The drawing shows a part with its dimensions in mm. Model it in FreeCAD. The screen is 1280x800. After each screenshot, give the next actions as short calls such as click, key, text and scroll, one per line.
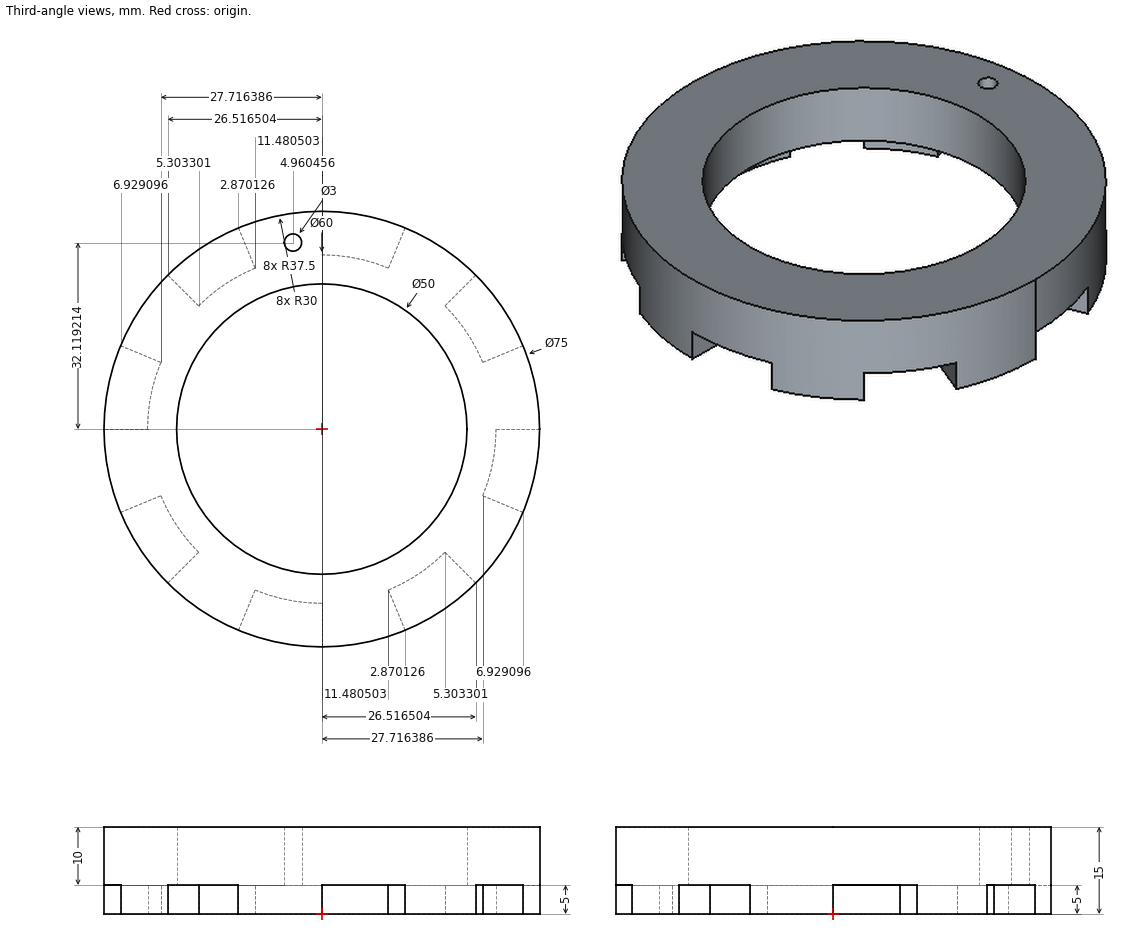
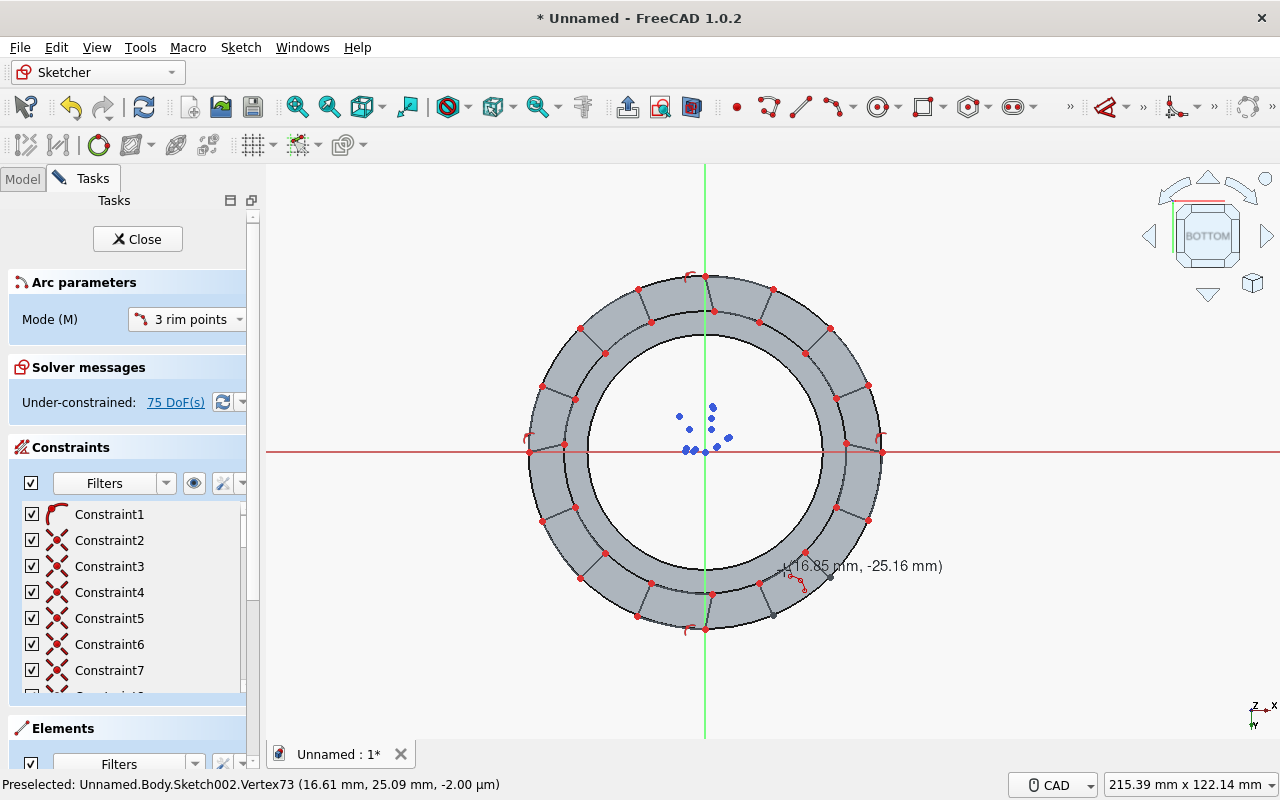
click(773, 616)
click(830, 578)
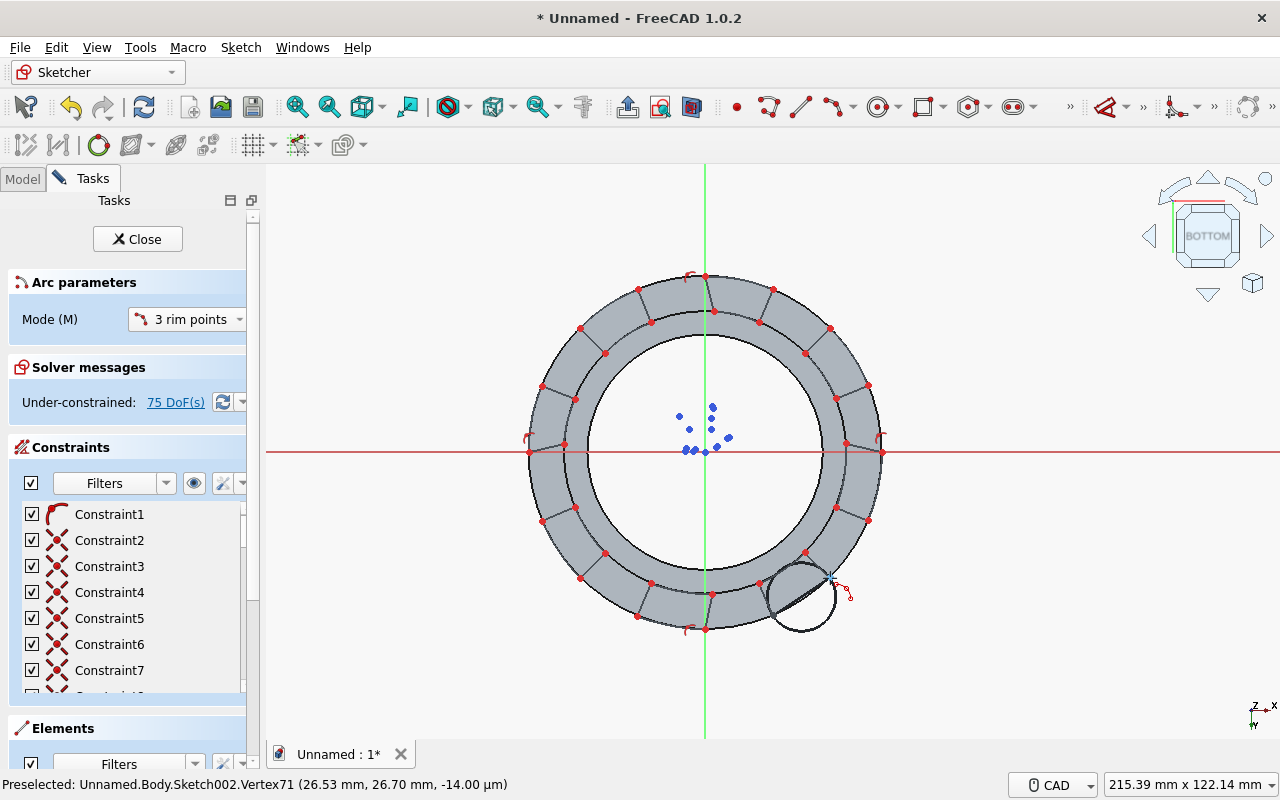
scroll(803, 599, up, 8)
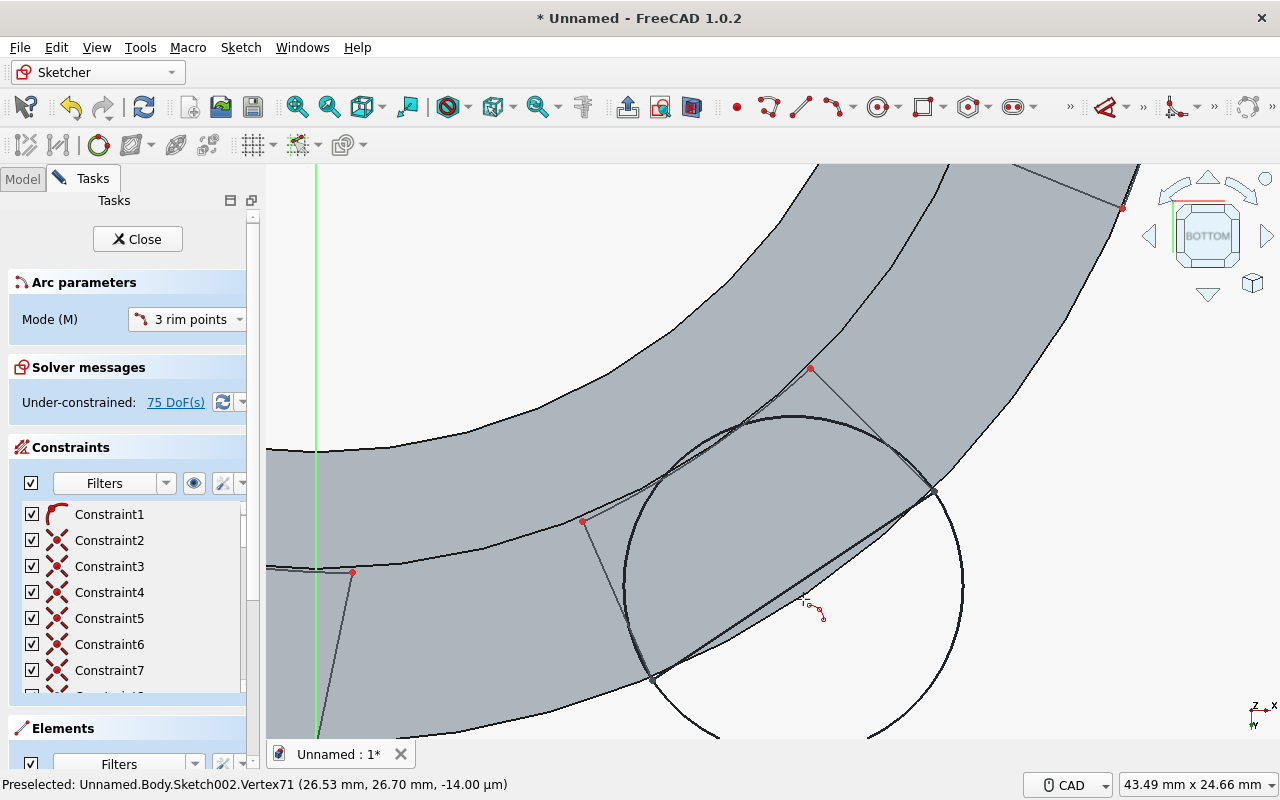
click(802, 596)
key(Escape)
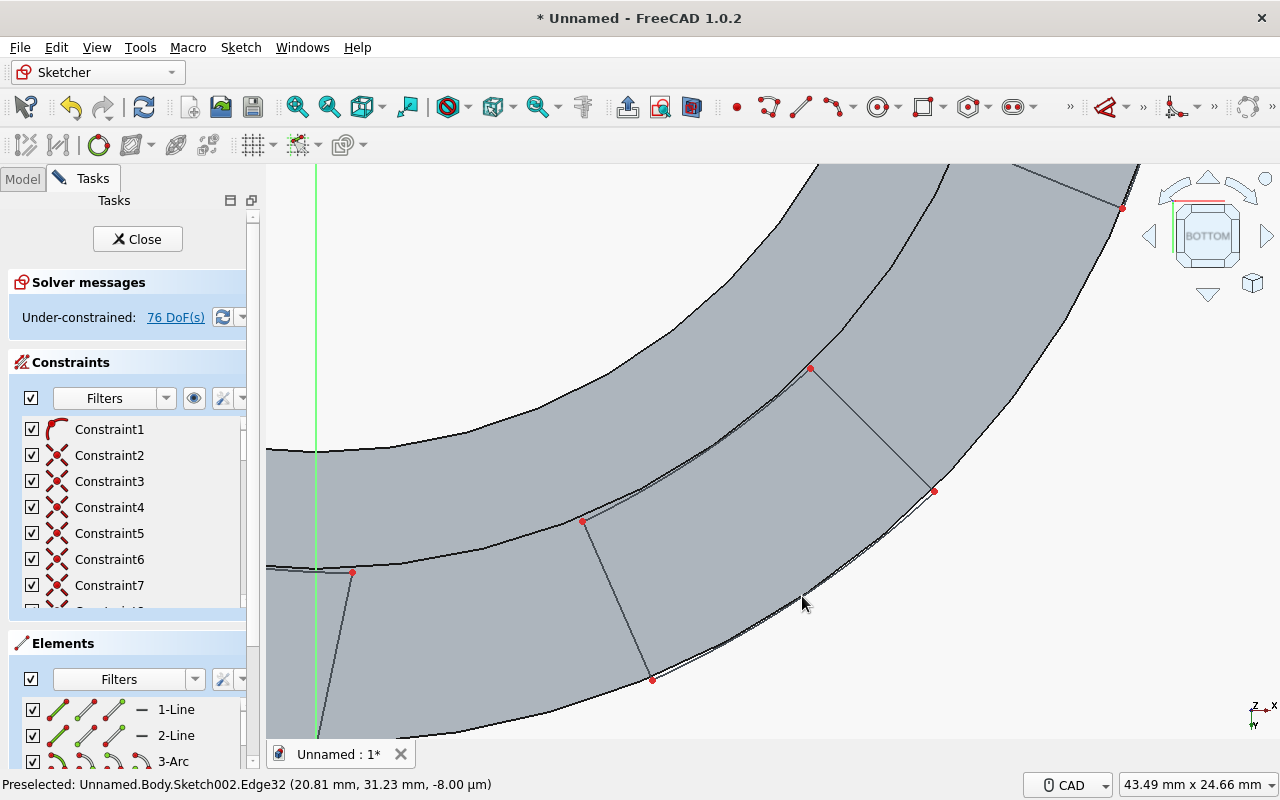
scroll(327, 695, up, 2)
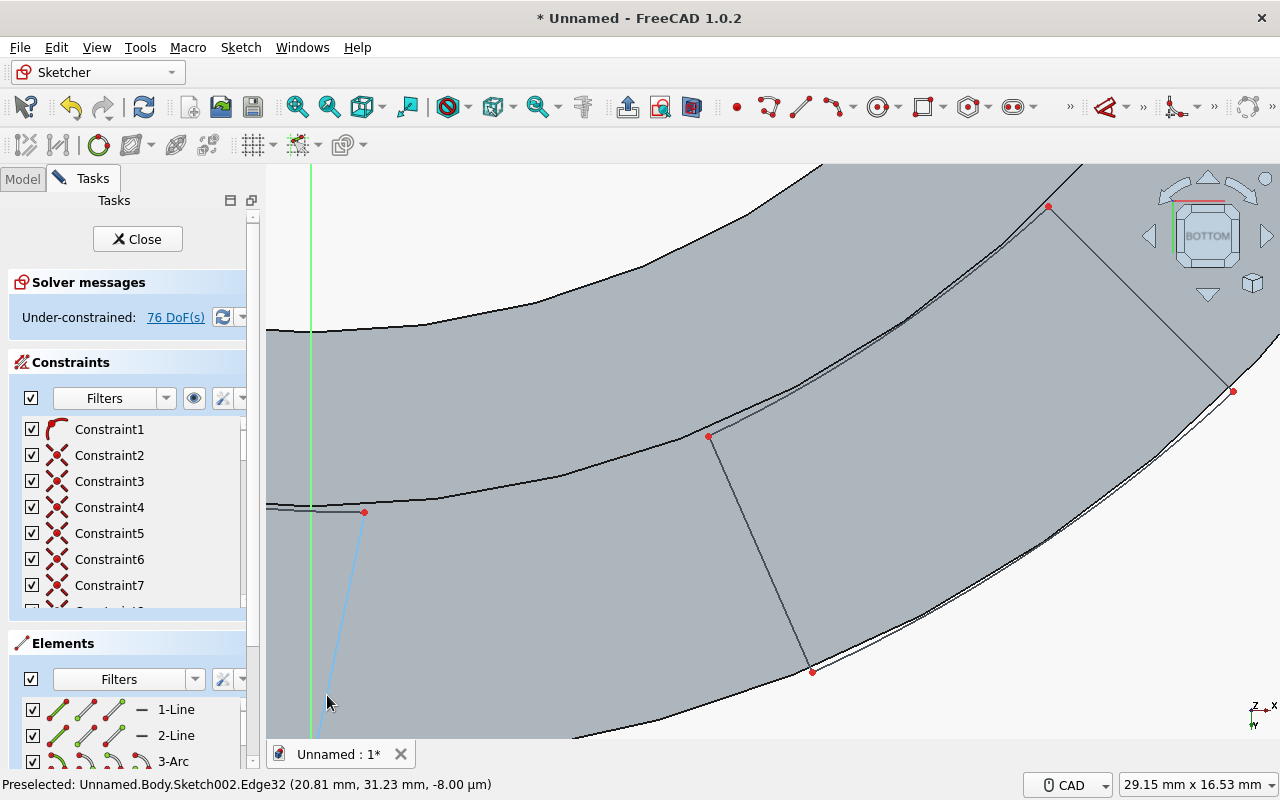
click(327, 695)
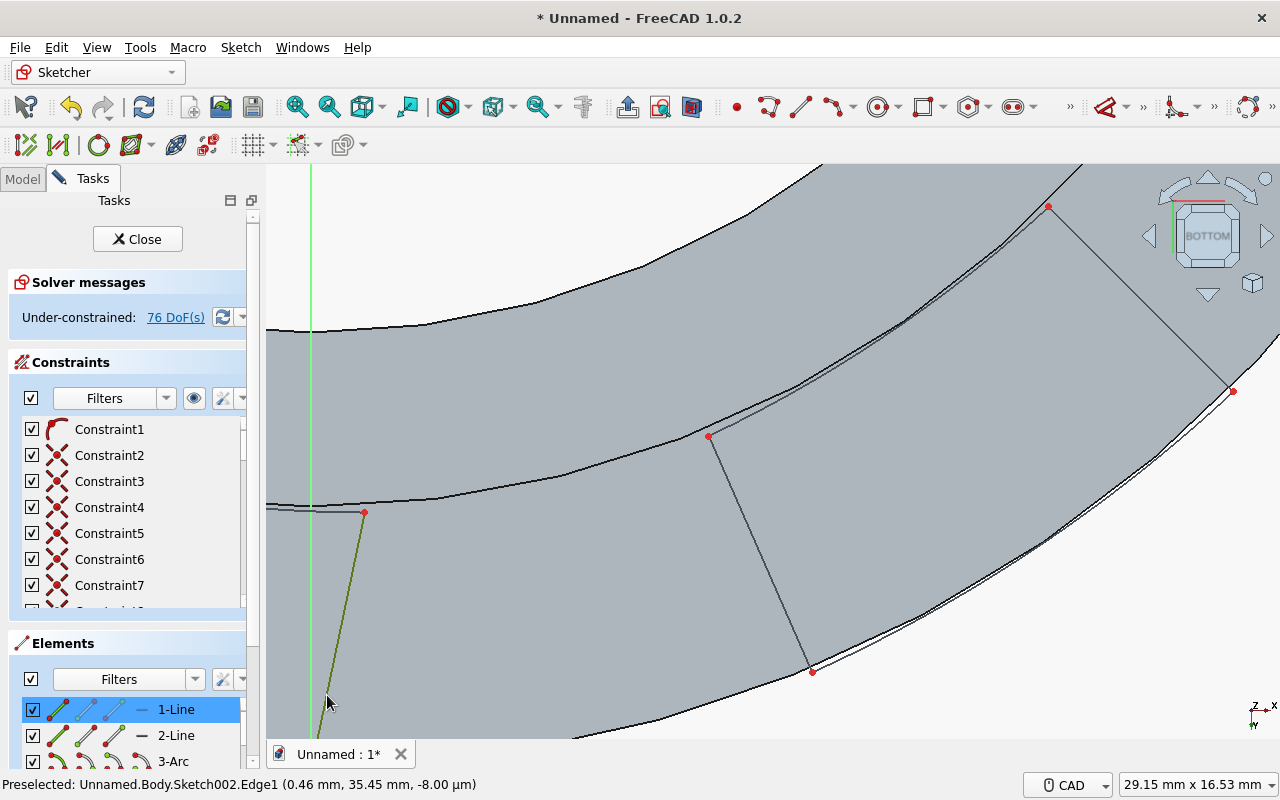
key(v)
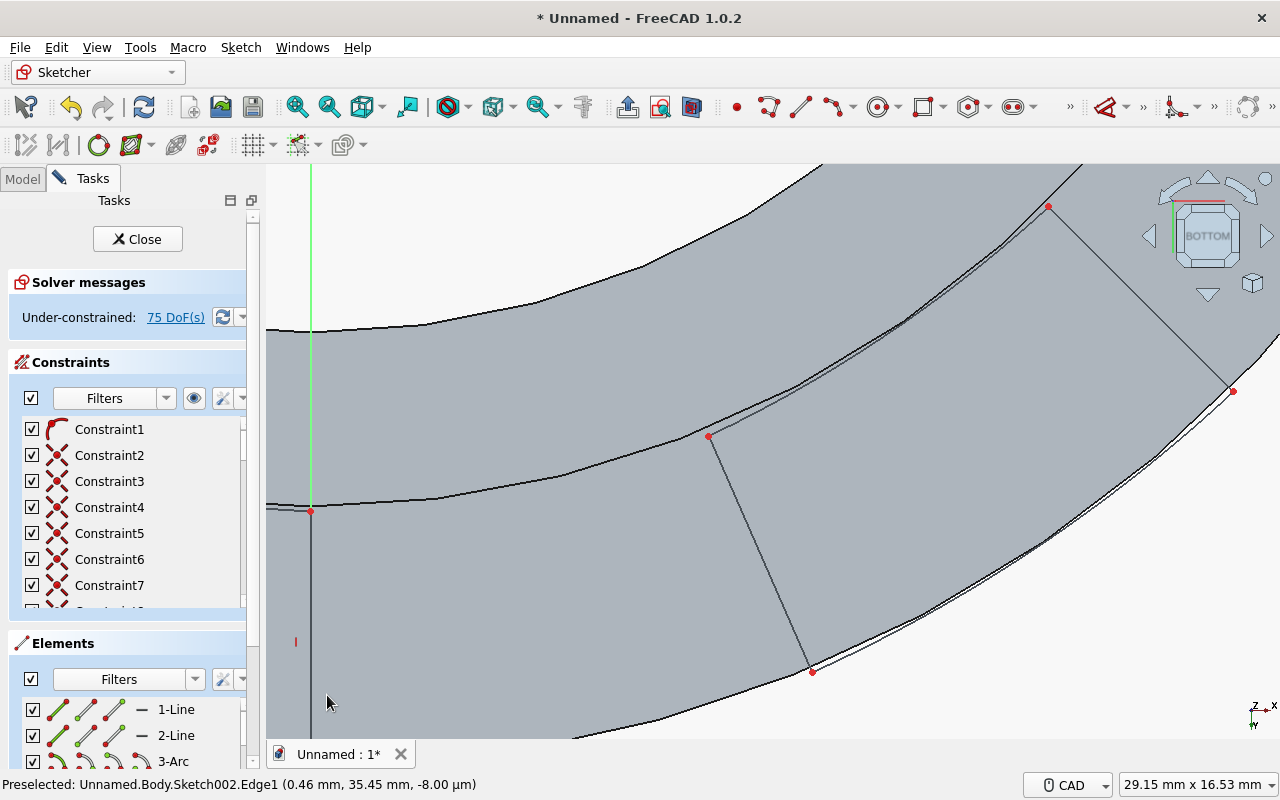
scroll(766, 606, down, 10)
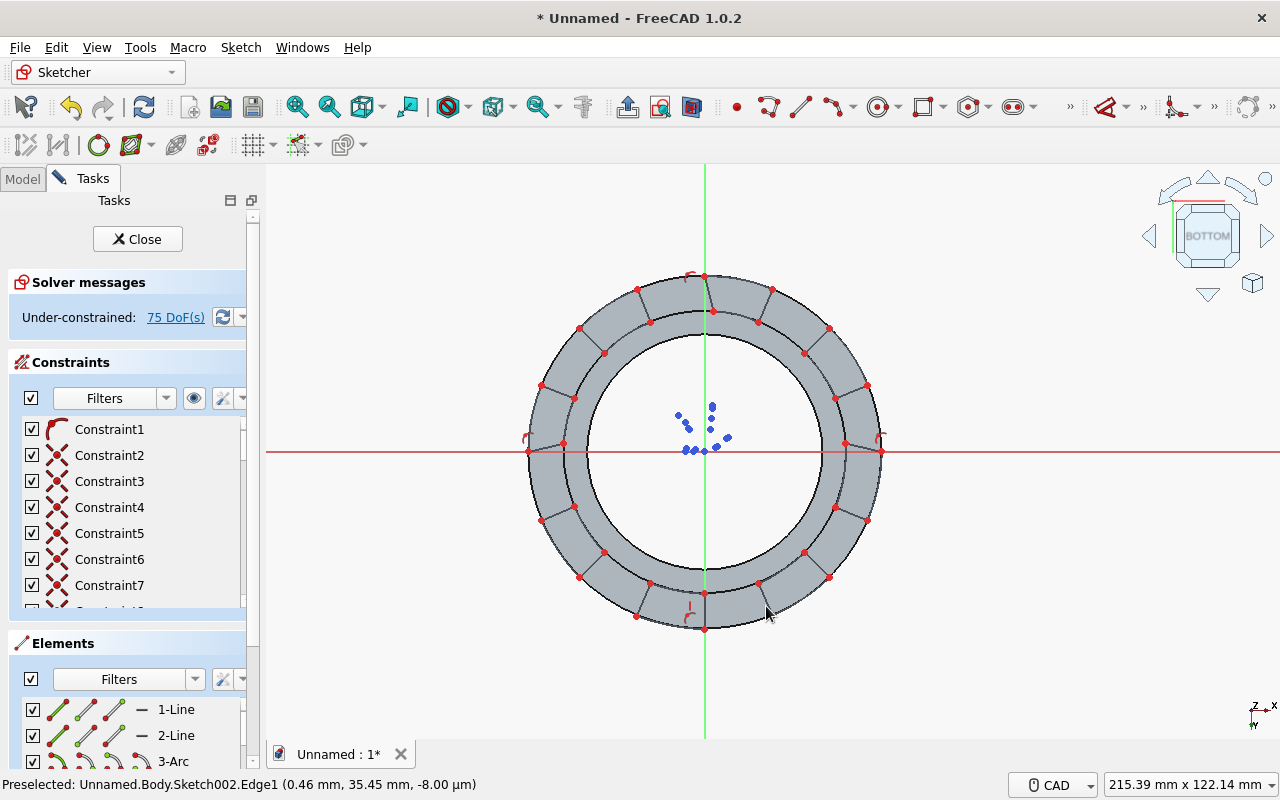
scroll(539, 449, up, 9)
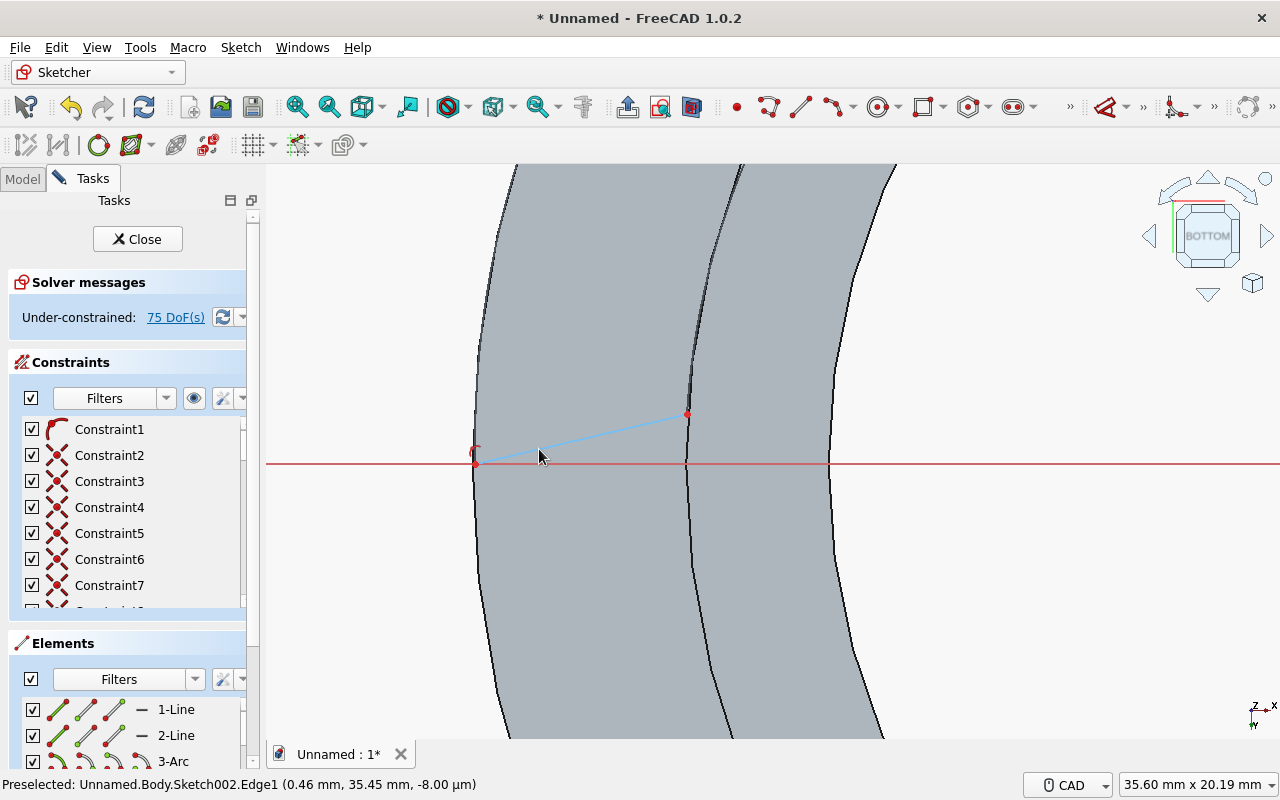
click(539, 449)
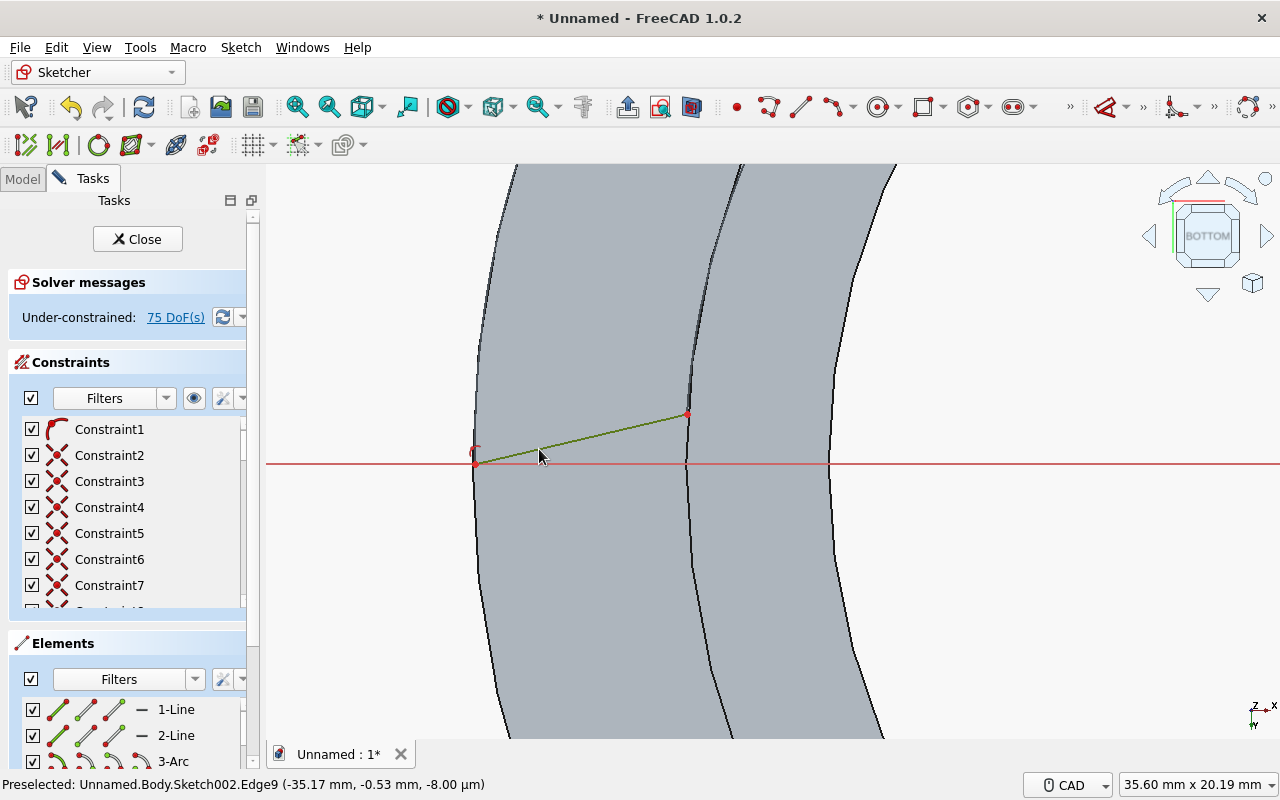
key(h)